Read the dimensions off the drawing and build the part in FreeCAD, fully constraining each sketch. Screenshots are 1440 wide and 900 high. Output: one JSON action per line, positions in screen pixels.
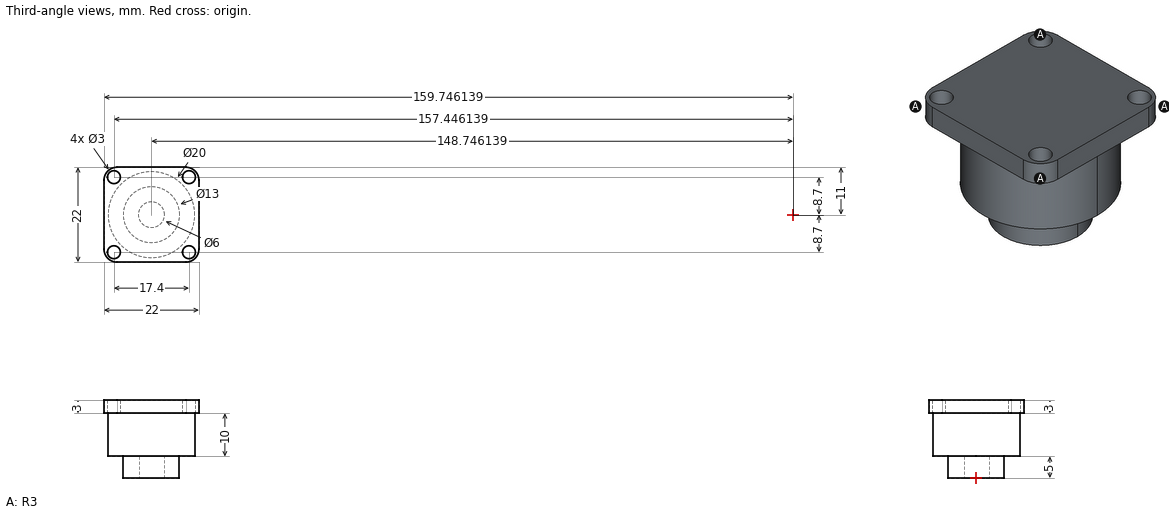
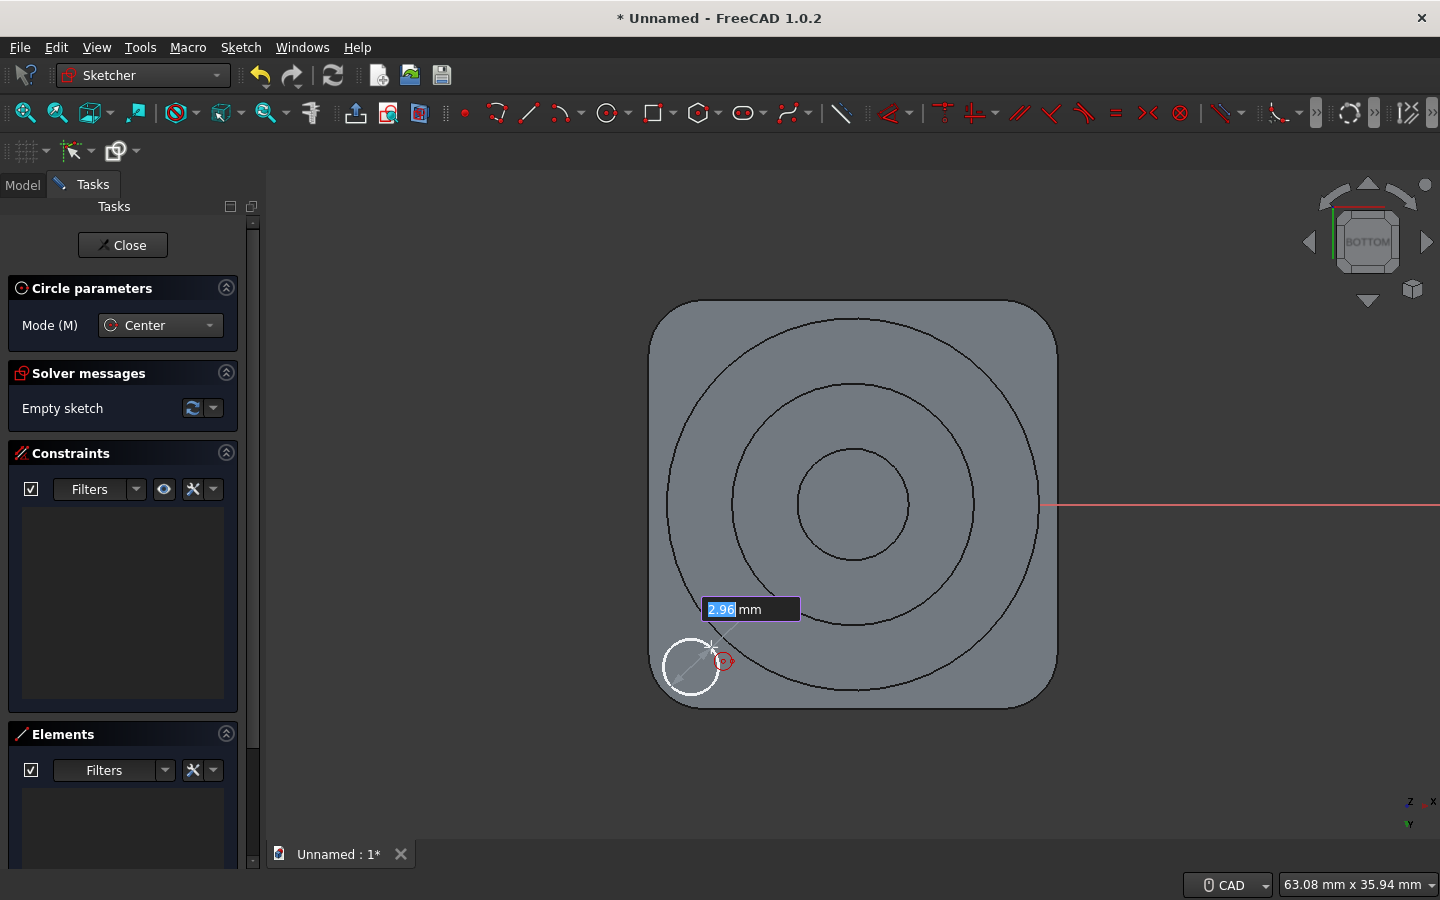
{"action": "type", "text": "3"}
{"action": "key", "text": "Return"}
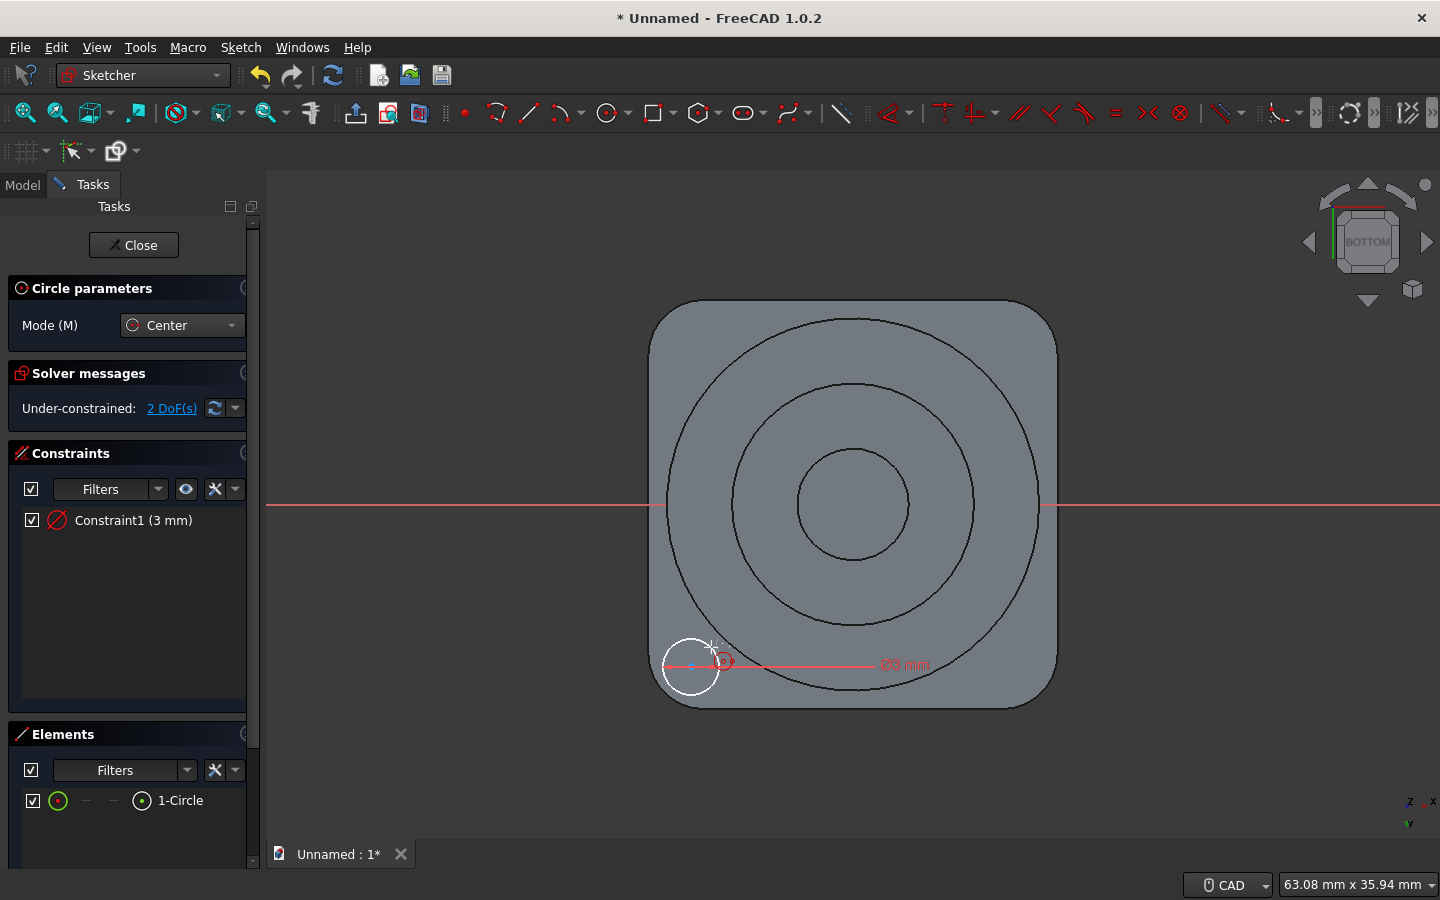
{"action": "left_click", "coordinate": [691, 343]}
{"action": "mouse_move", "coordinate": [711, 323]}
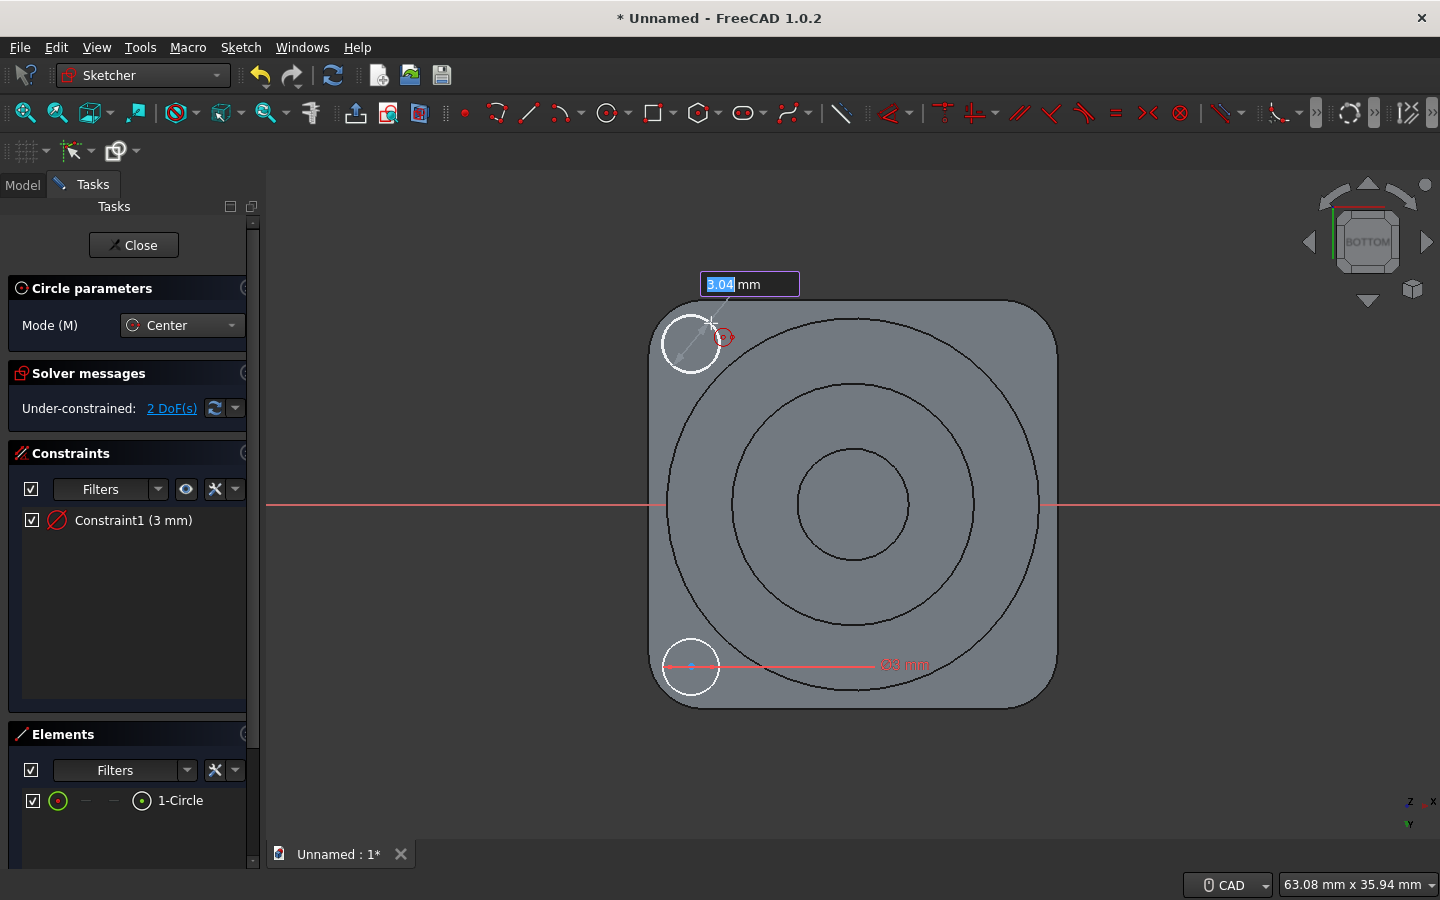
{"action": "type", "text": "3"}
{"action": "key", "text": "Return"}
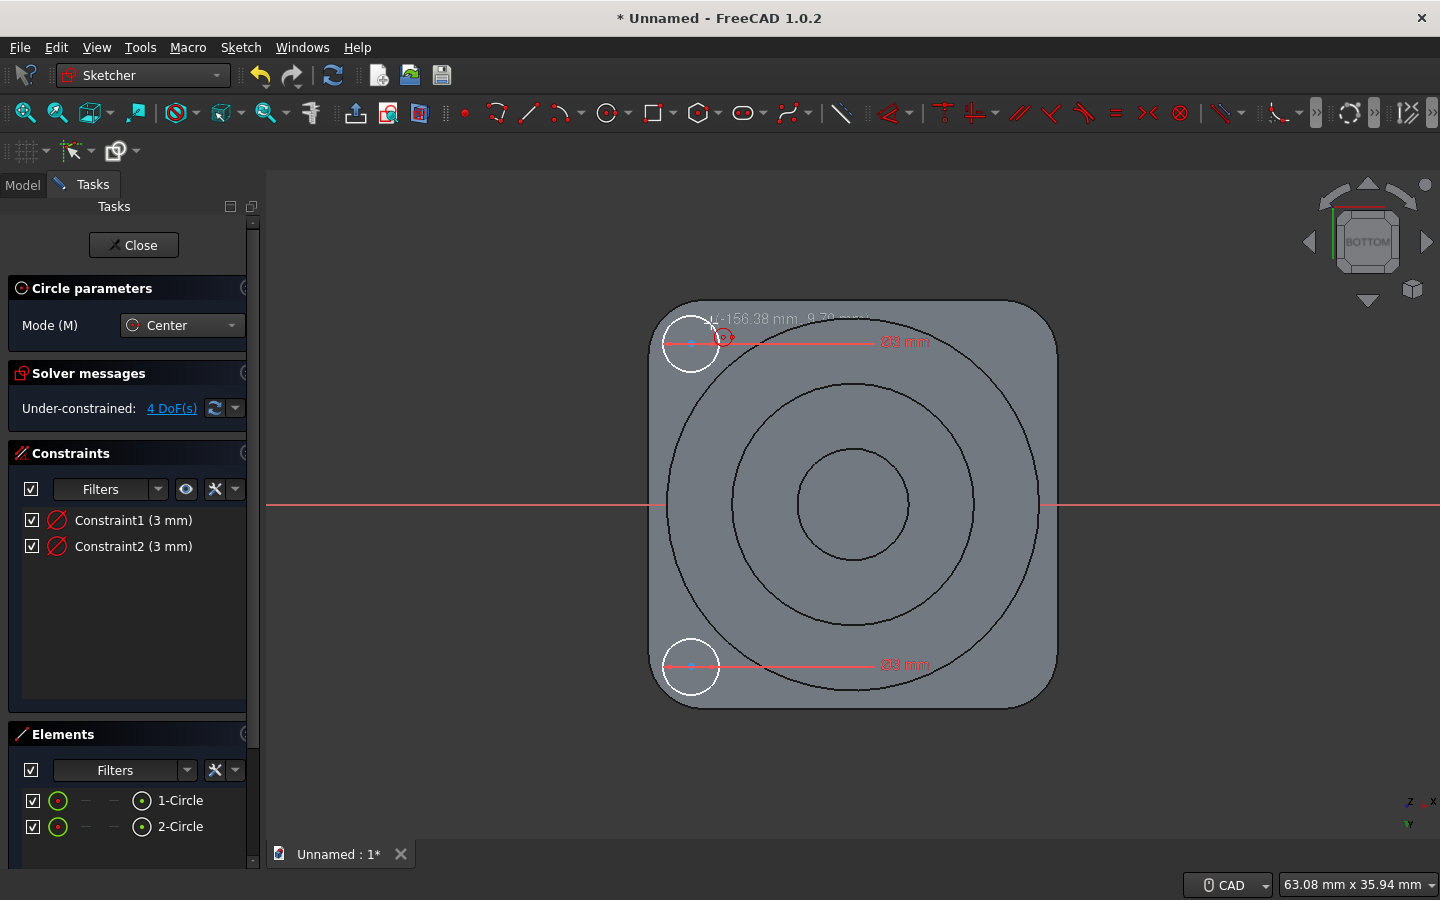
{"action": "left_click", "coordinate": [1015, 343]}
{"action": "mouse_move", "coordinate": [1035, 323]}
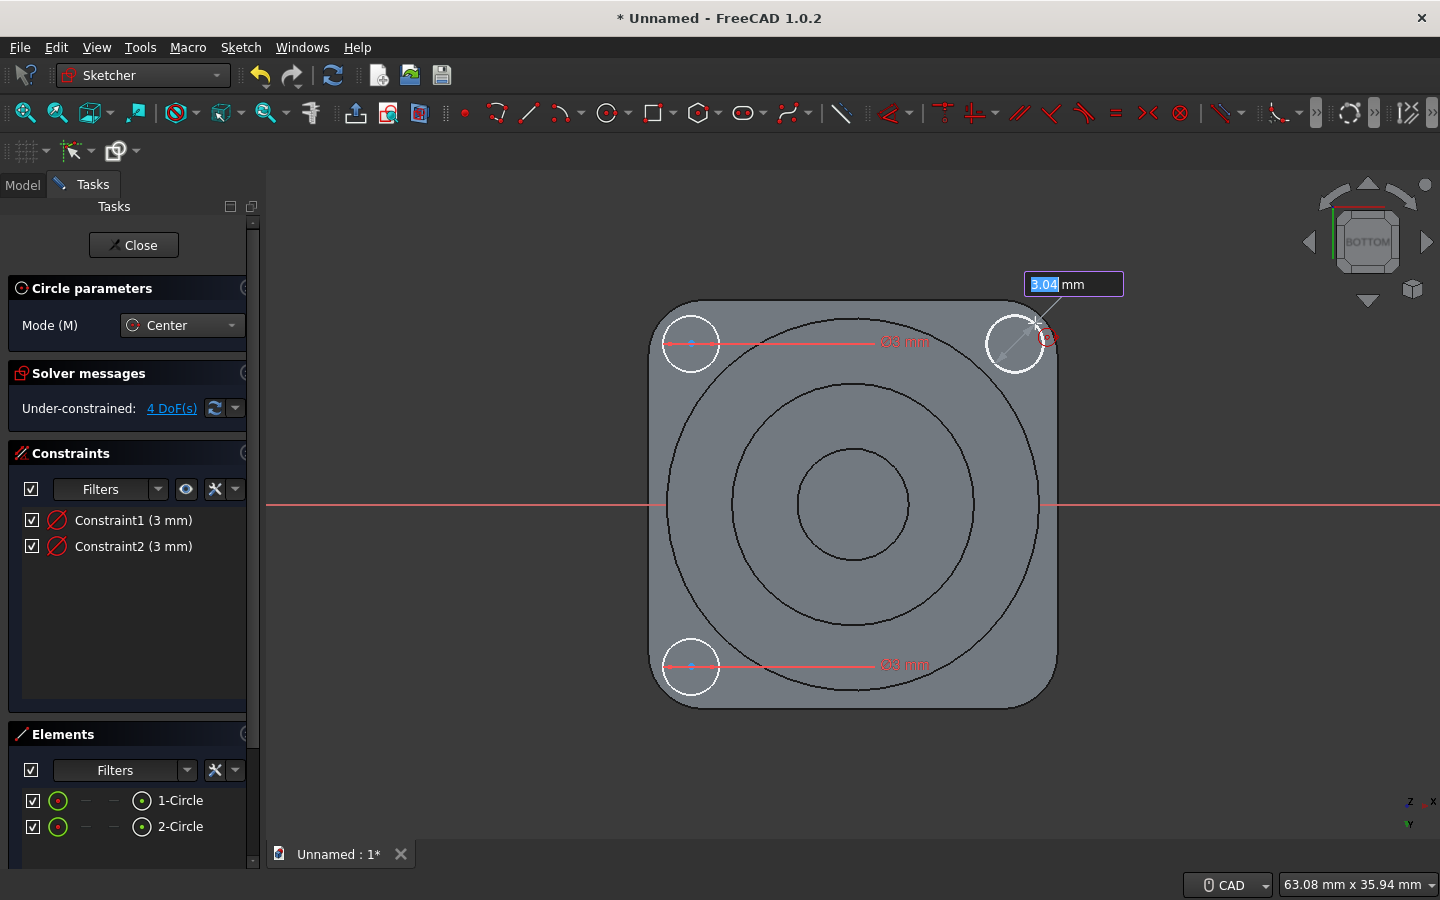
{"action": "type", "text": "3"}
{"action": "key", "text": "Return"}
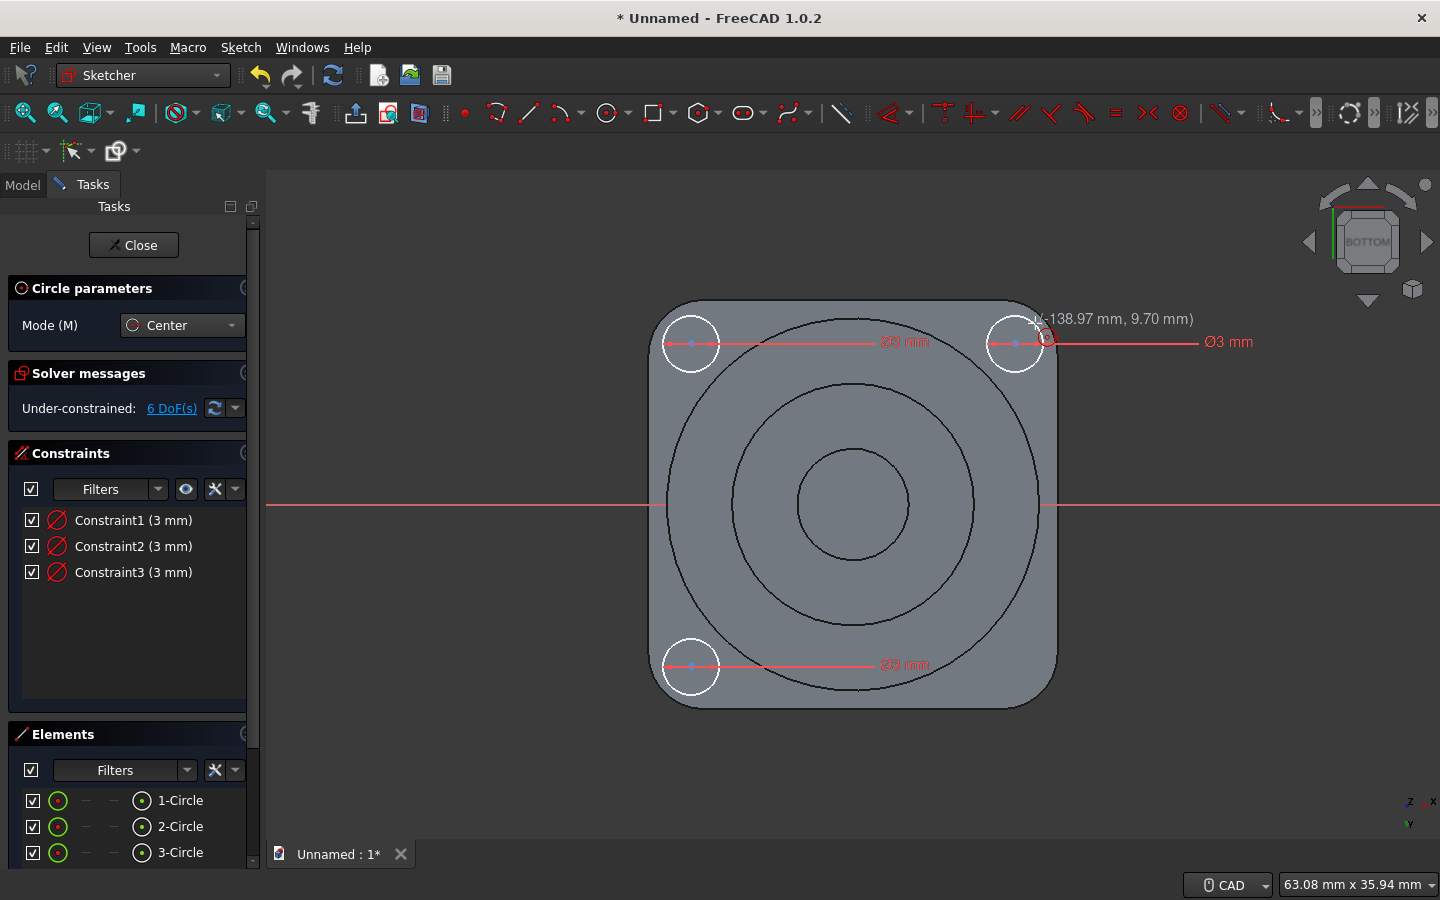
{"action": "left_click", "coordinate": [1015, 666]}
{"action": "mouse_move", "coordinate": [1035, 647]}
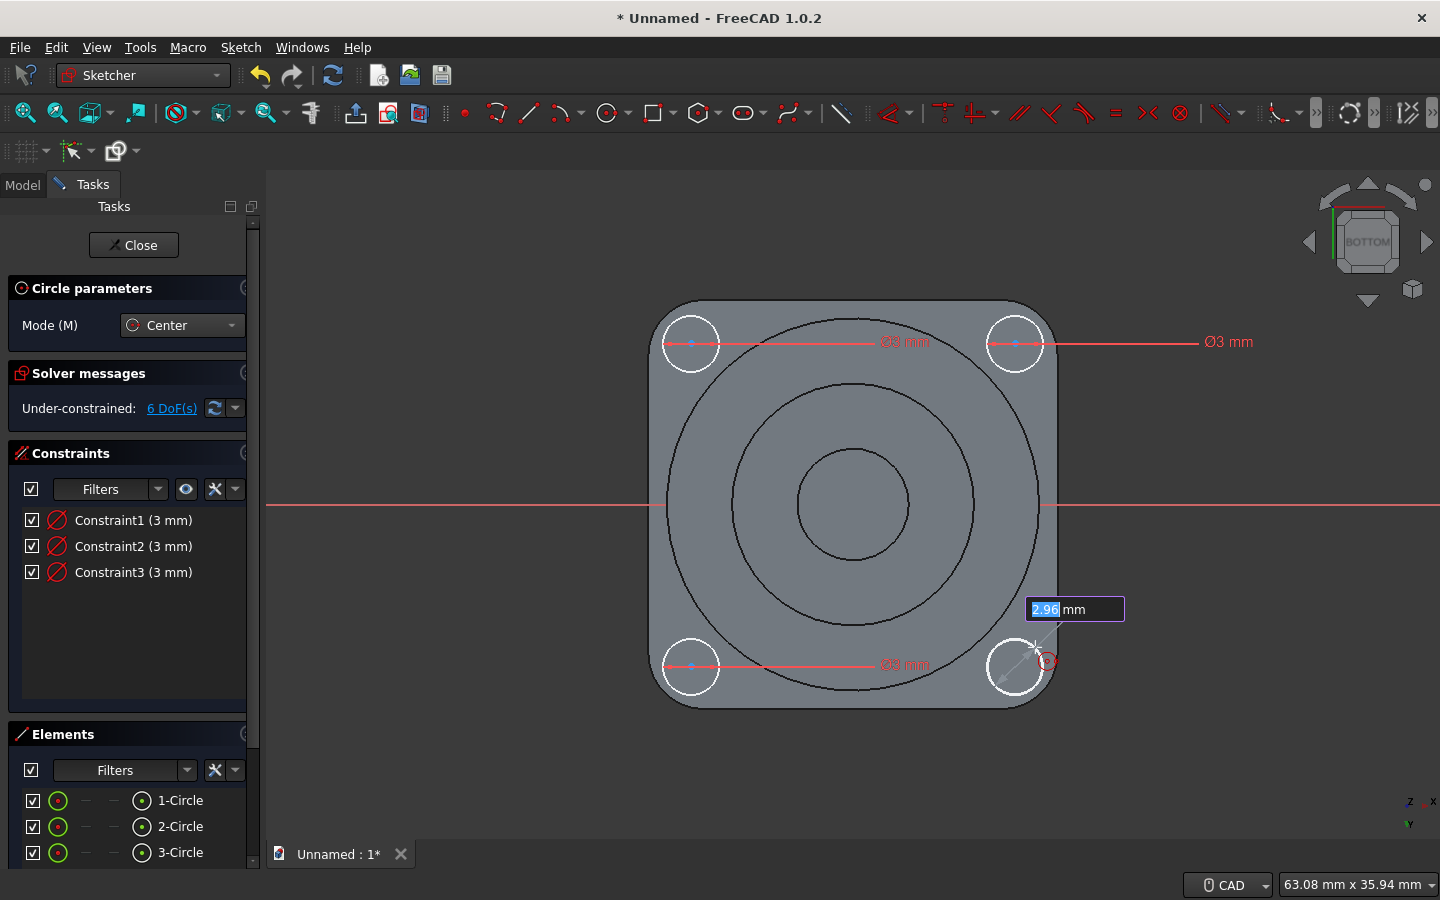
{"action": "type", "text": "3"}
{"action": "key", "text": "Return"}
{"action": "key", "text": "Escape"}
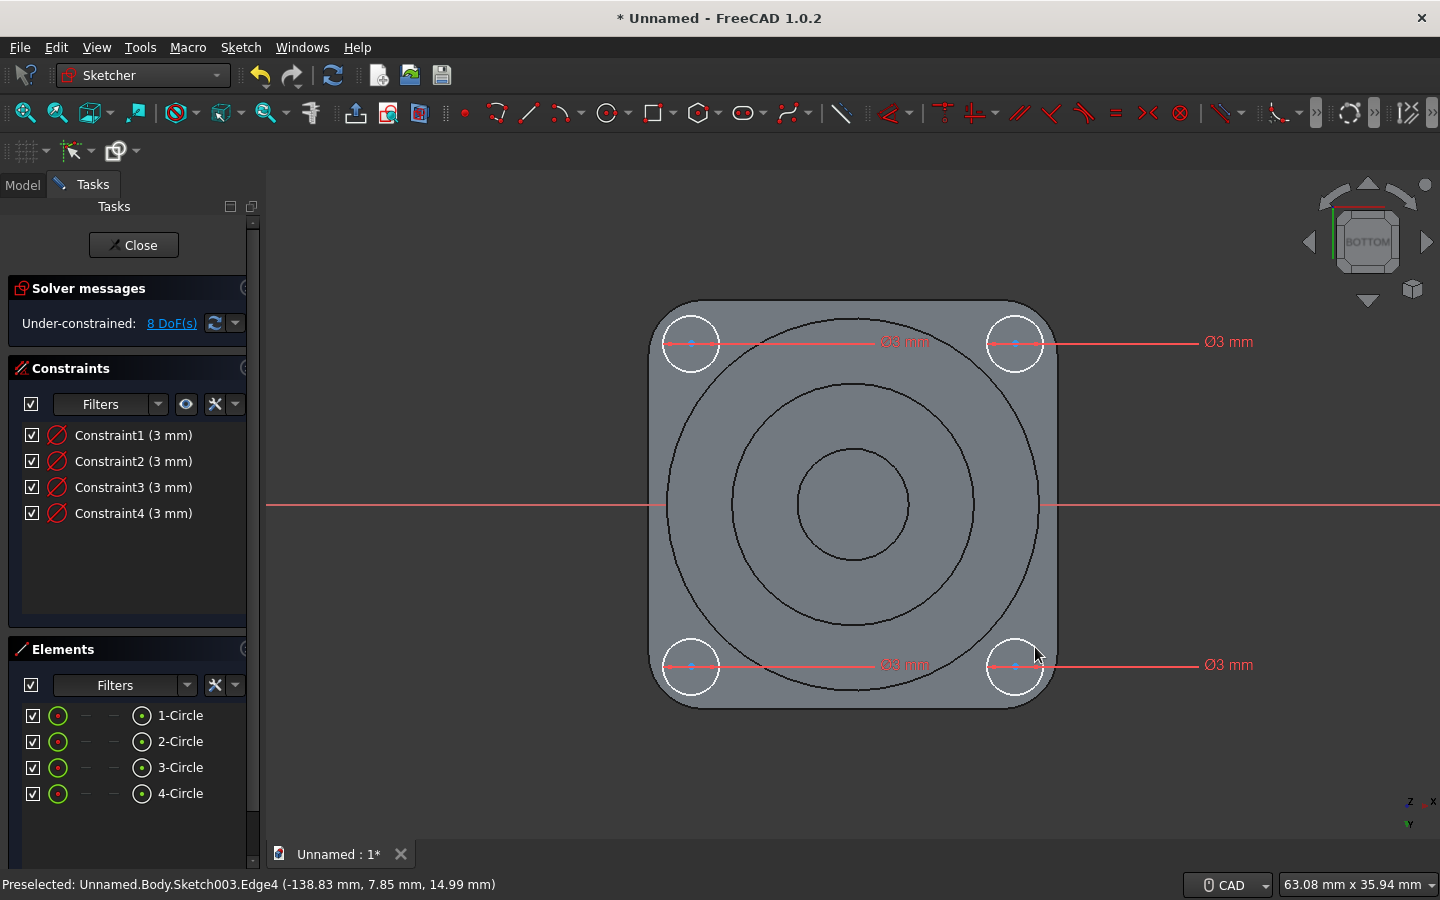
{"action": "left_click", "coordinate": [691, 667]}